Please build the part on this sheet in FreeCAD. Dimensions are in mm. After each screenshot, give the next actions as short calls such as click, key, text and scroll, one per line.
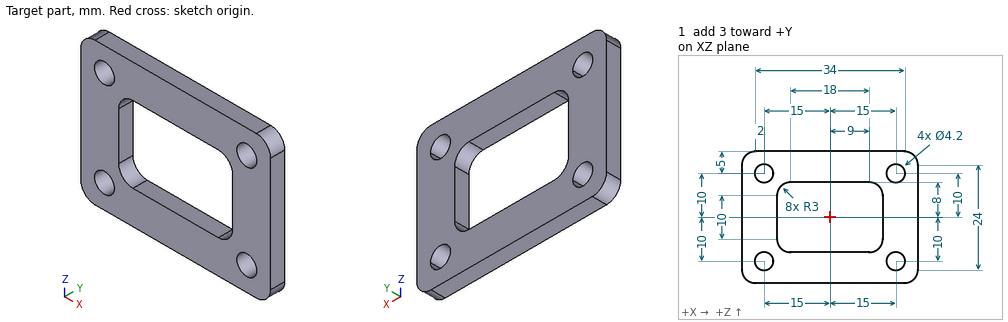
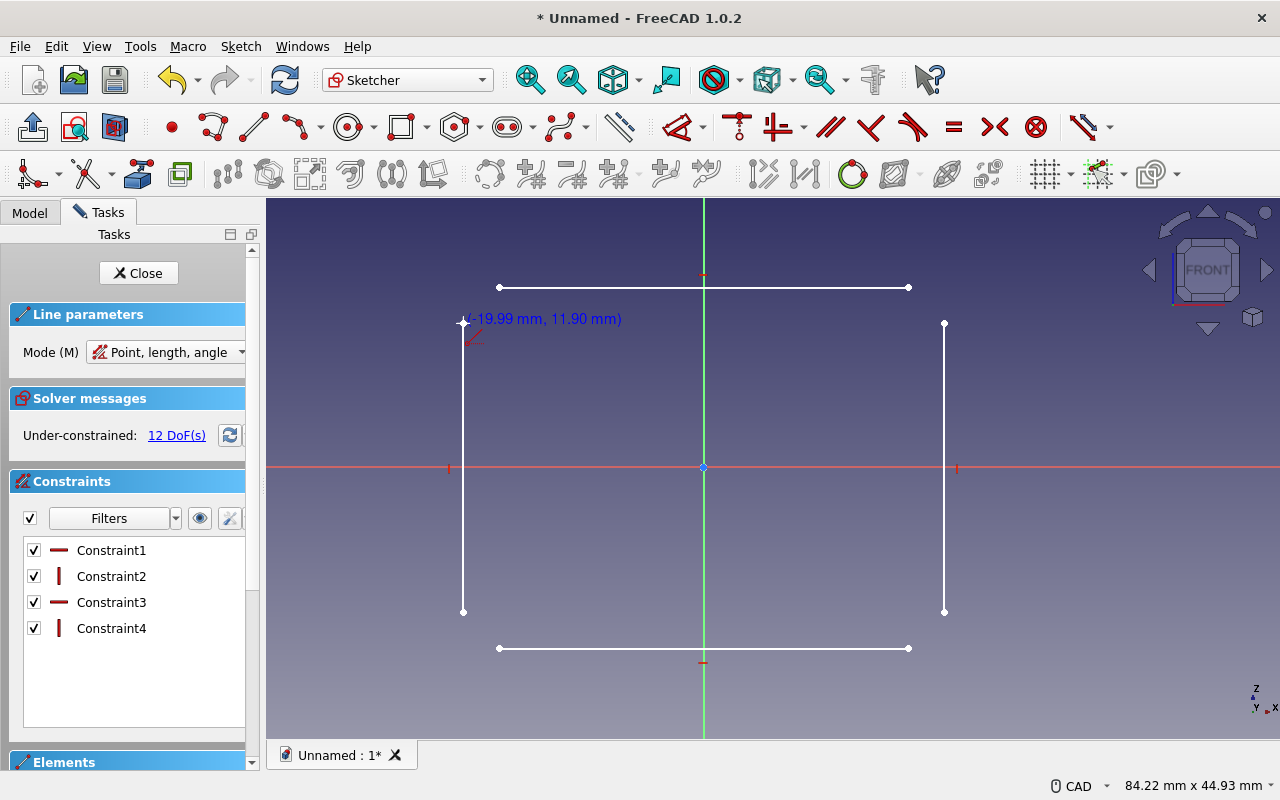
key(g)
key(3)
key(a)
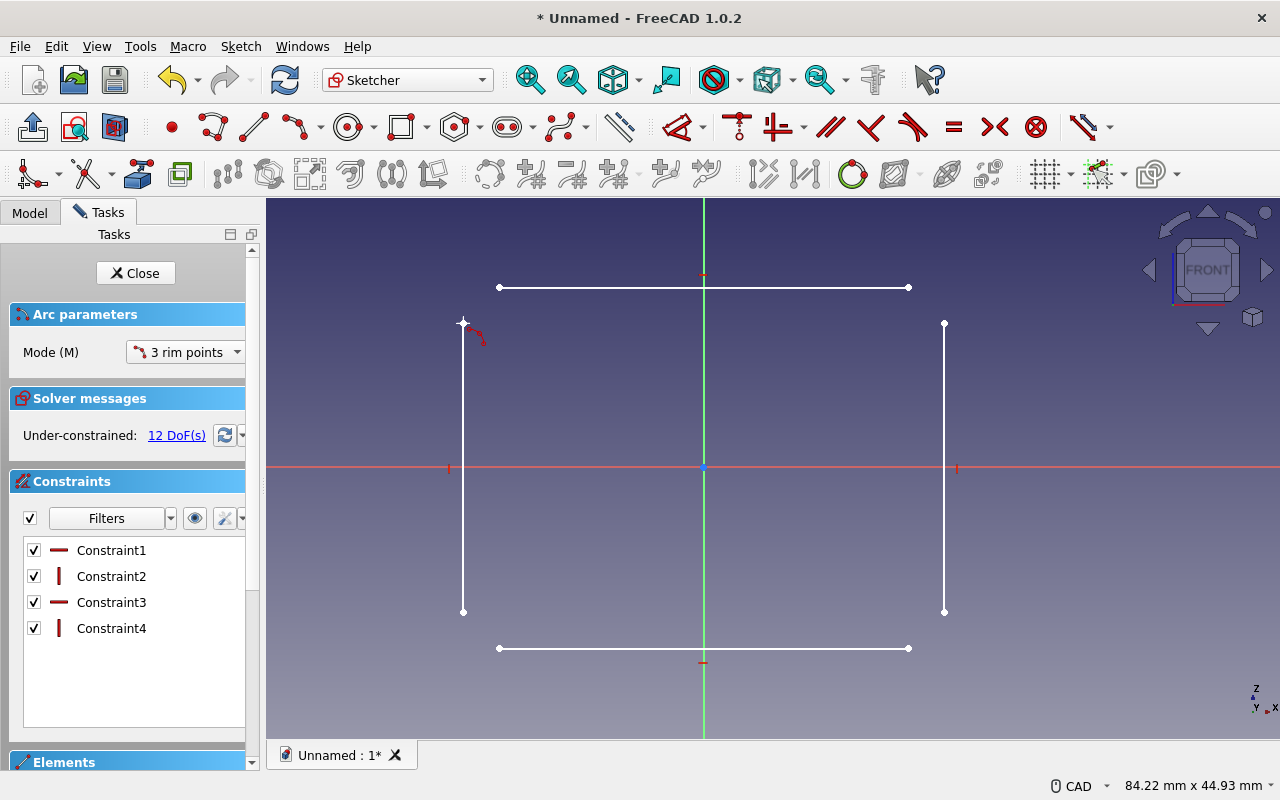
click(908, 288)
click(944, 324)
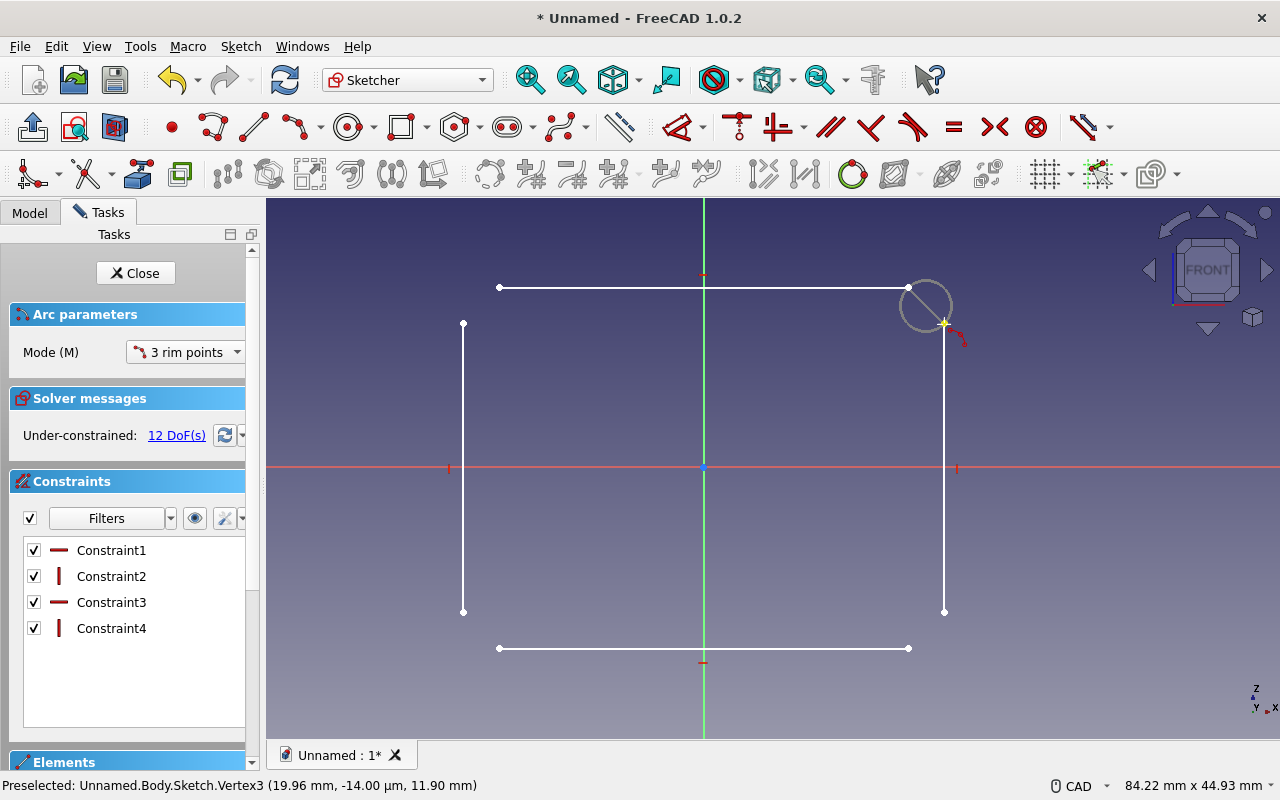
scroll(934, 297, up, 3)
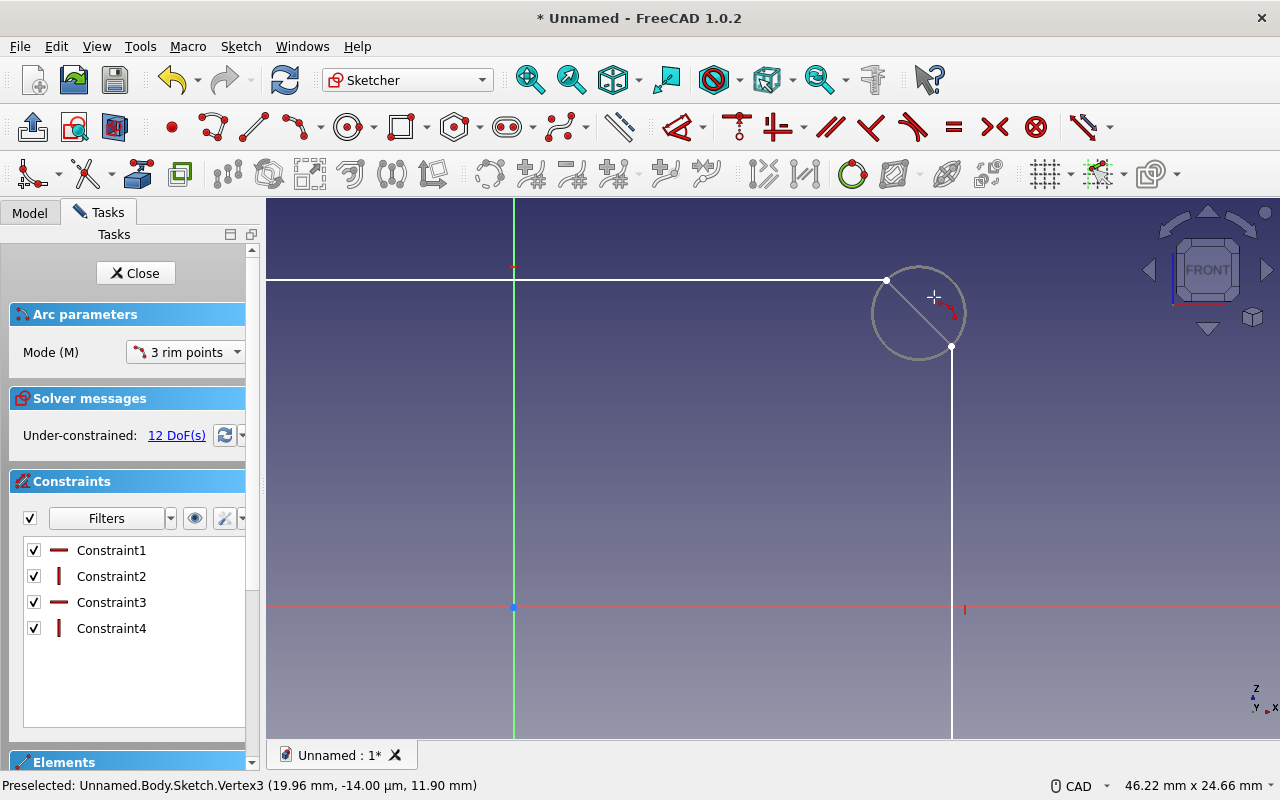
click(933, 297)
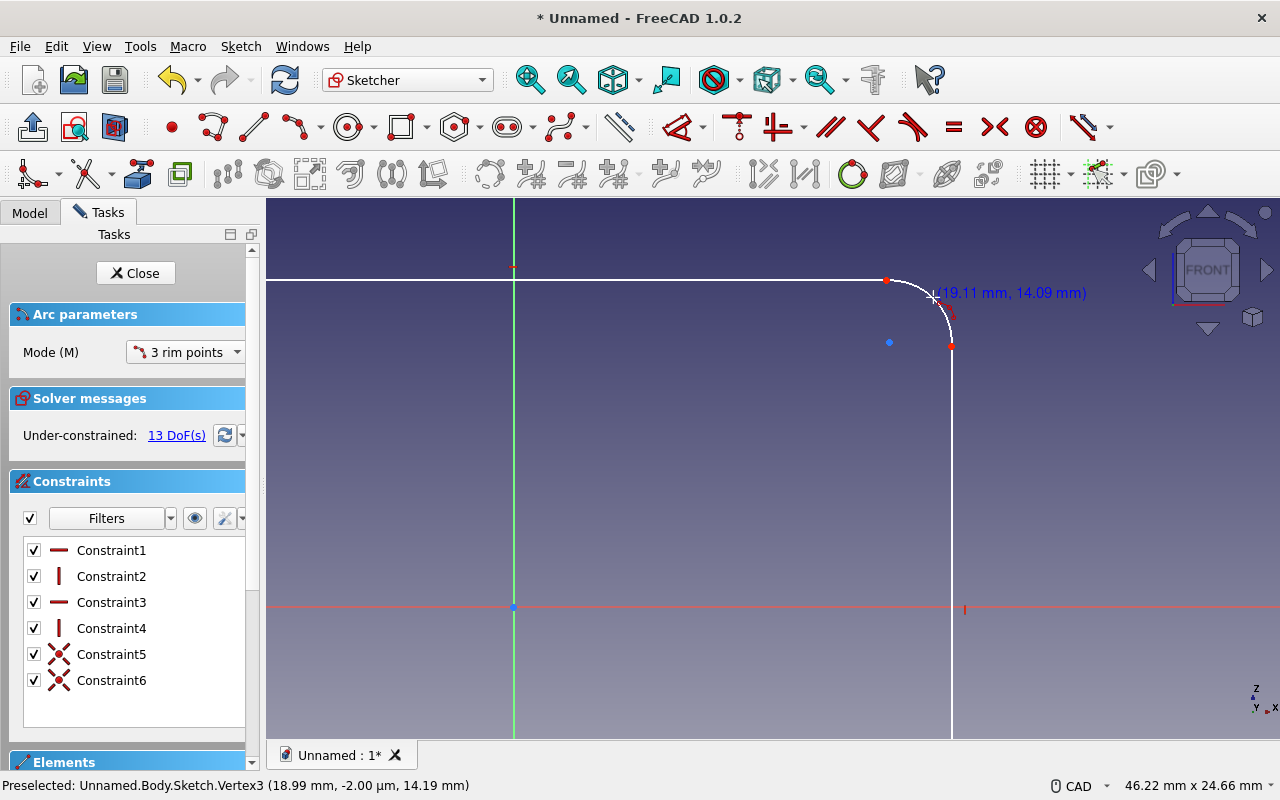
scroll(936, 300, down, 3)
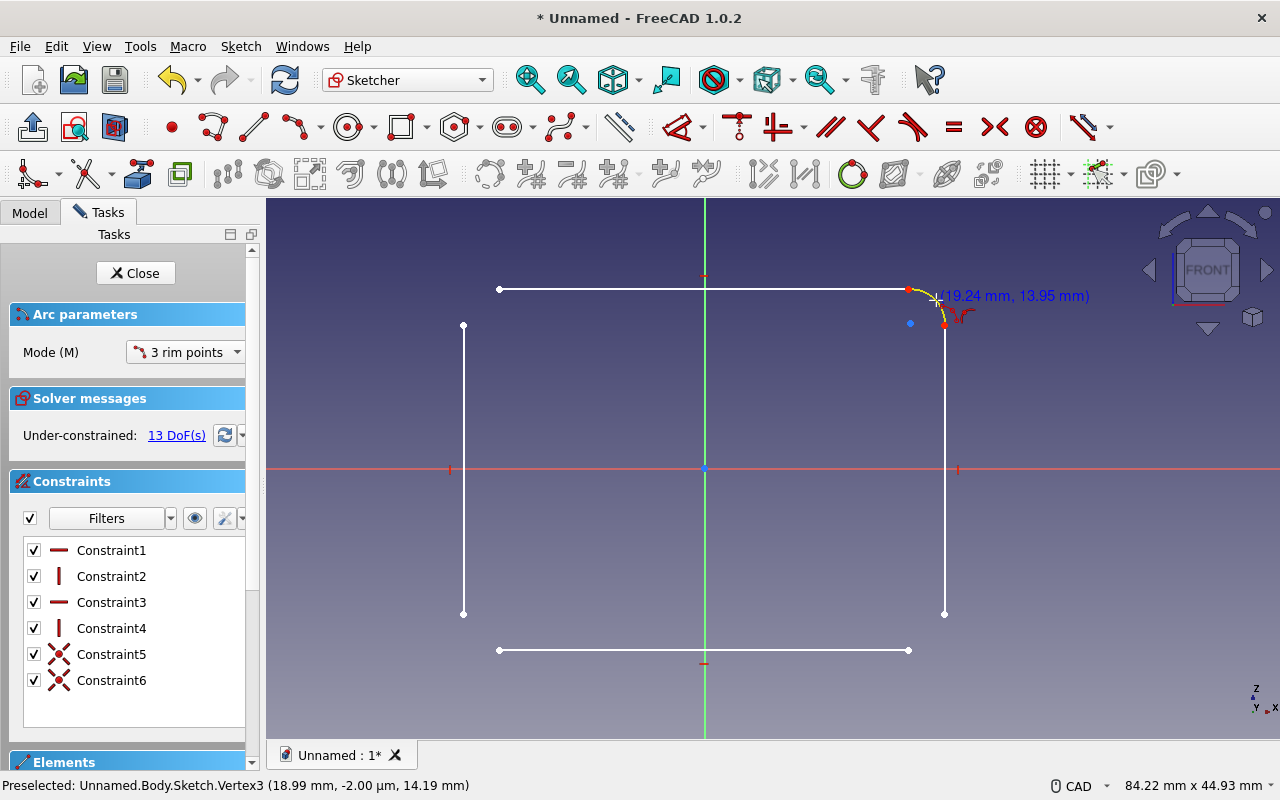
click(945, 614)
click(909, 650)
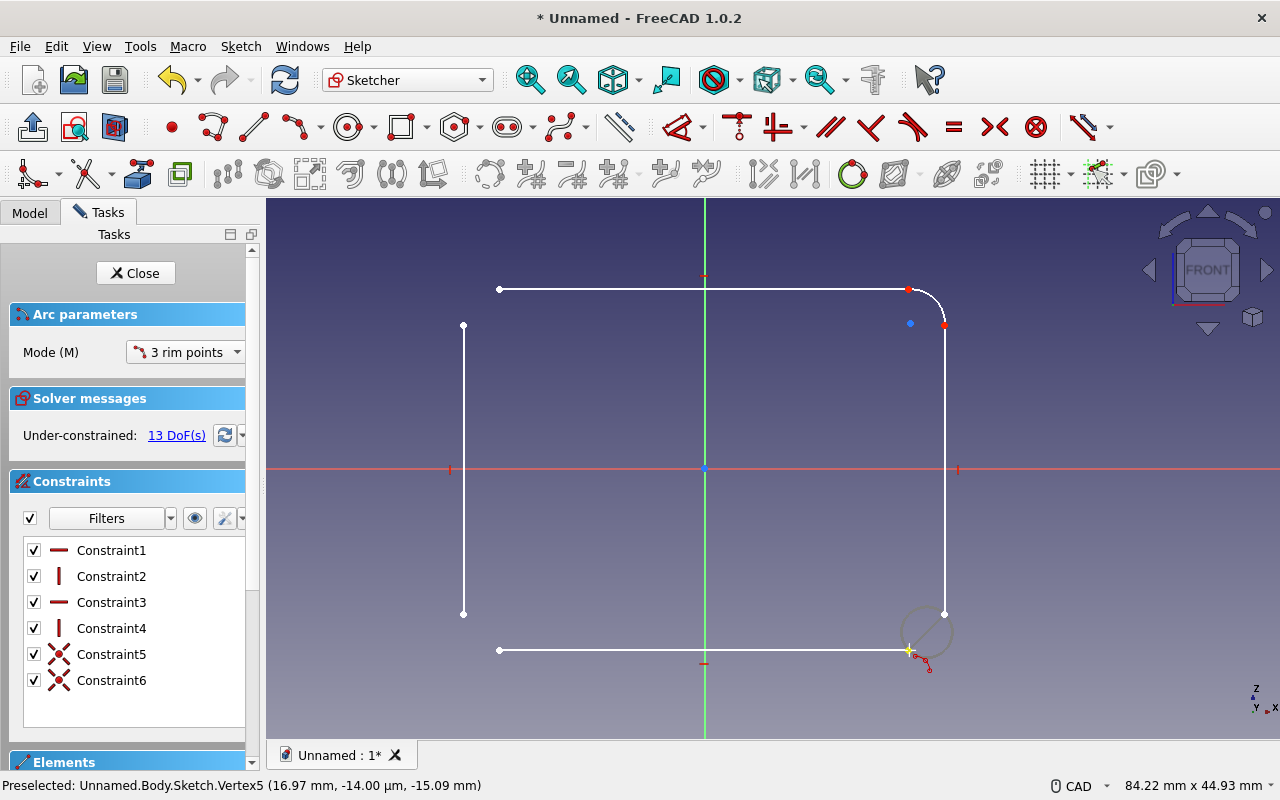
scroll(935, 639, up, 3)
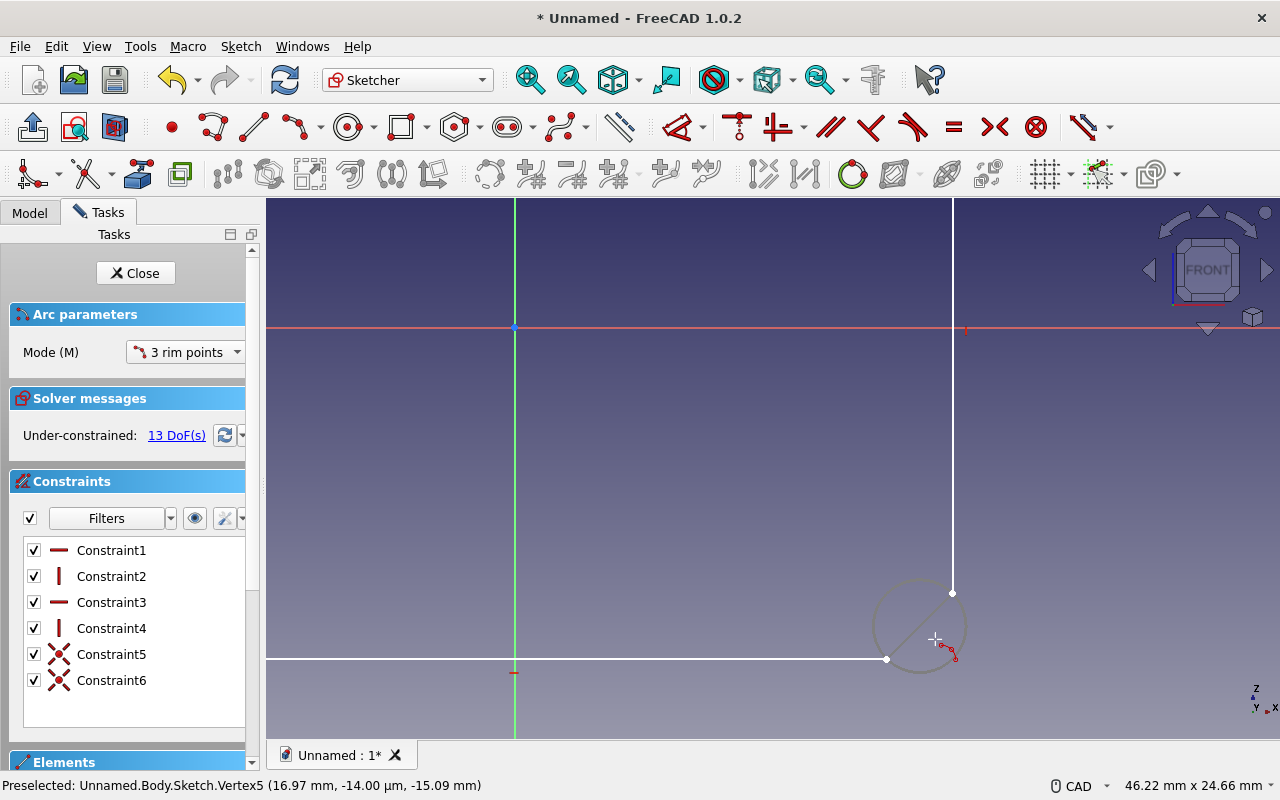
click(934, 638)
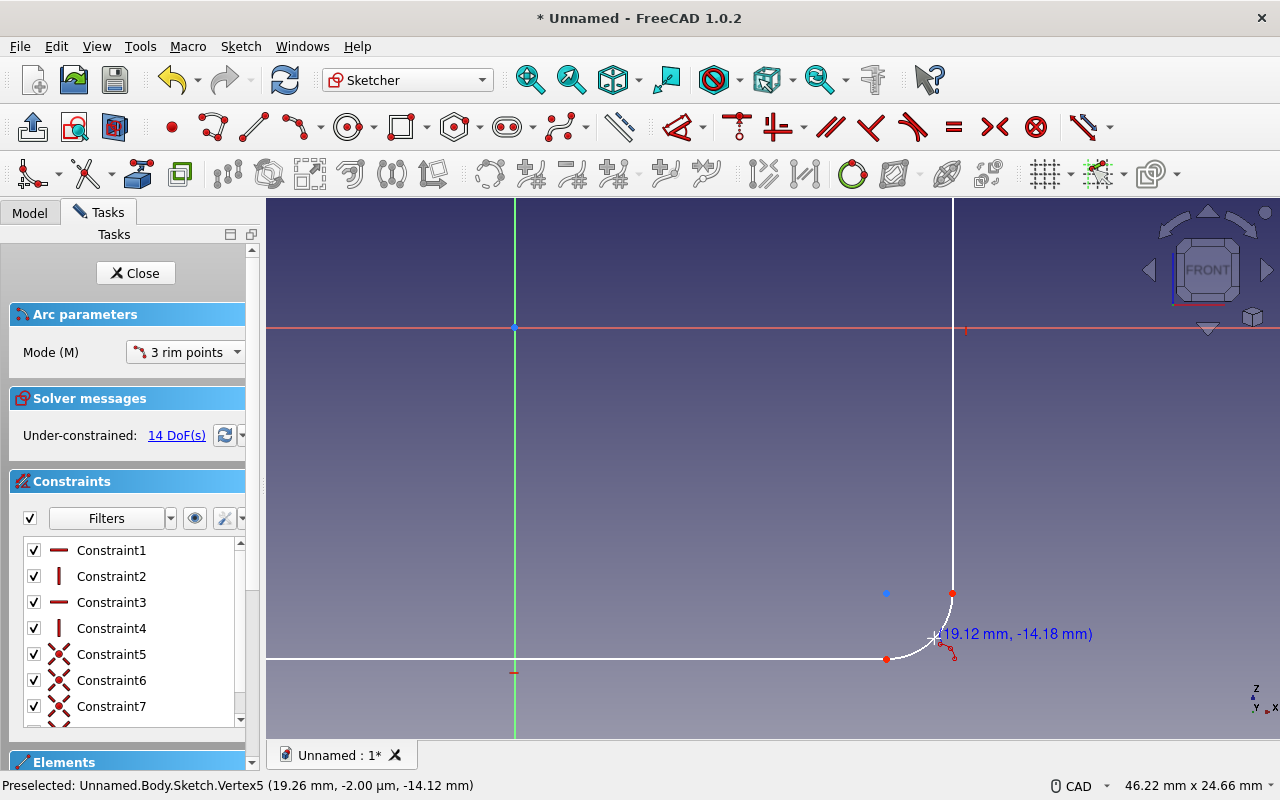
scroll(935, 640, down, 3)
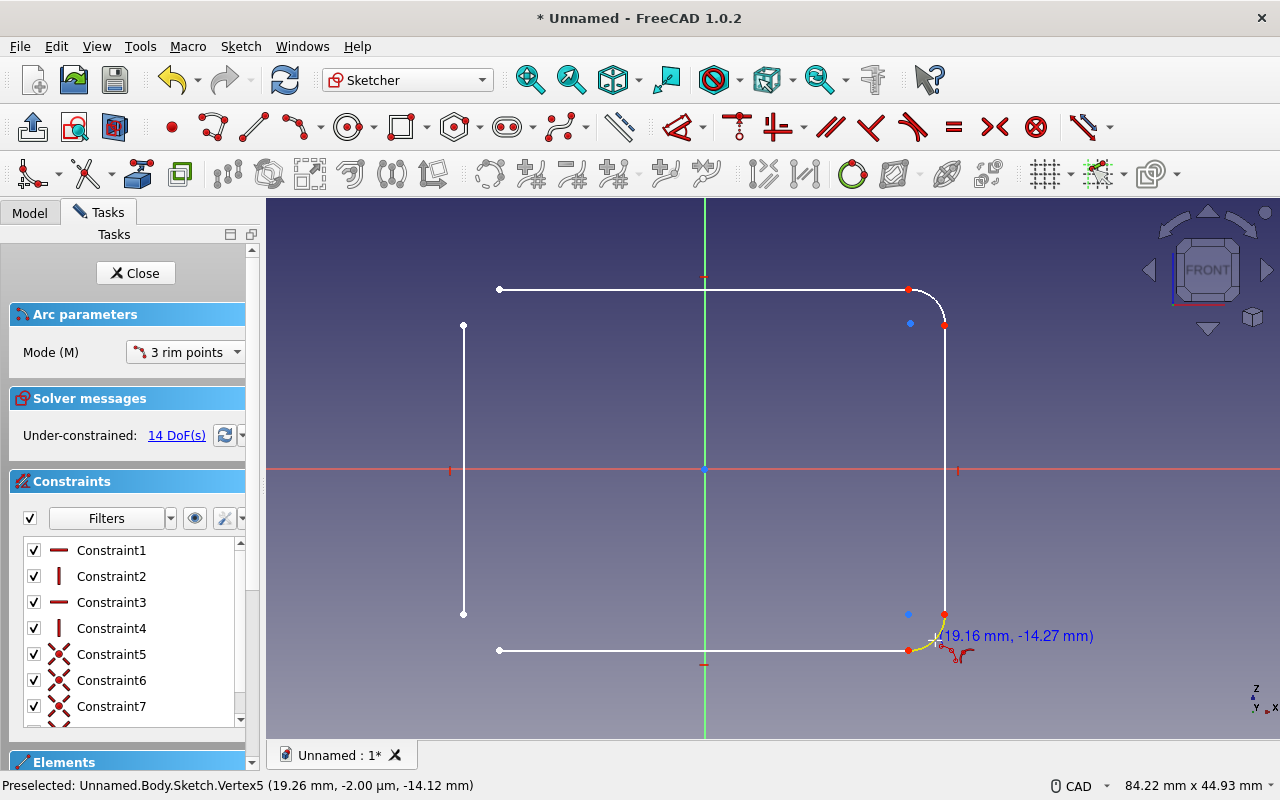
click(500, 651)
click(464, 615)